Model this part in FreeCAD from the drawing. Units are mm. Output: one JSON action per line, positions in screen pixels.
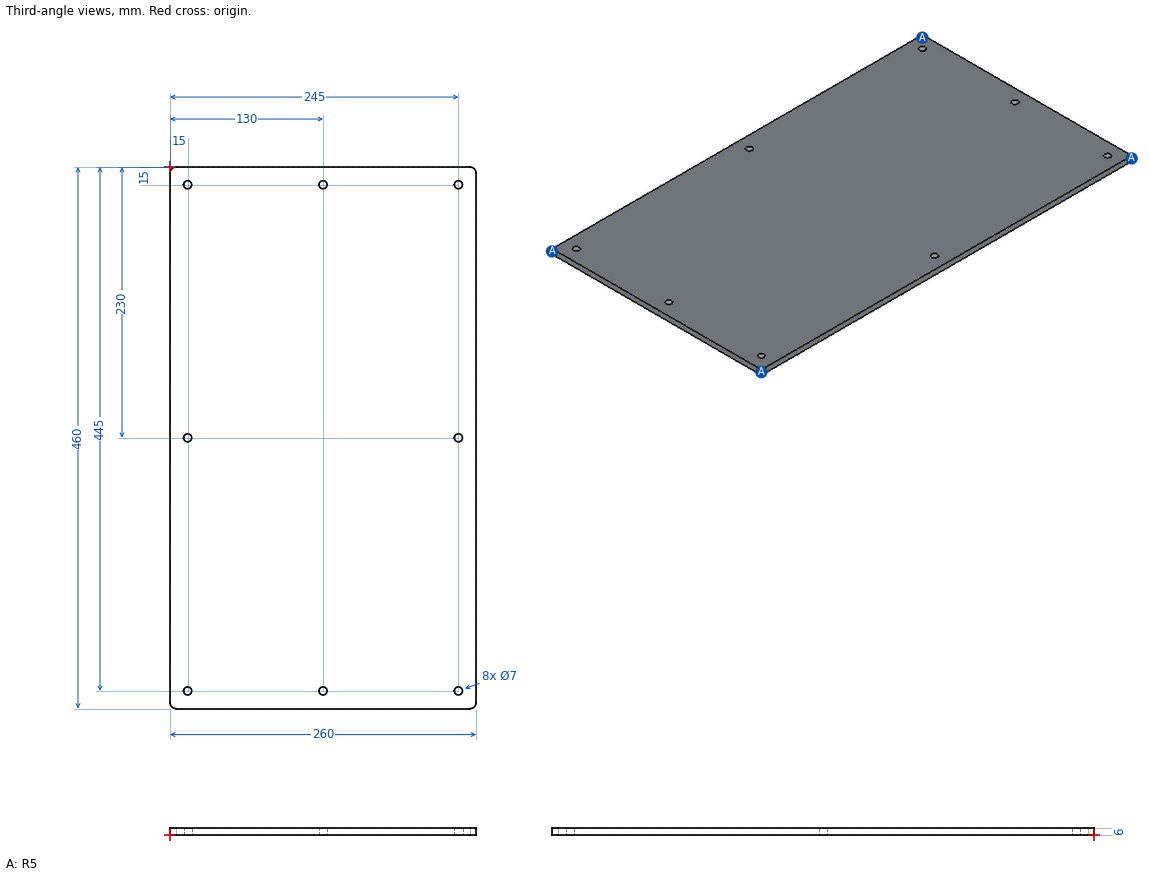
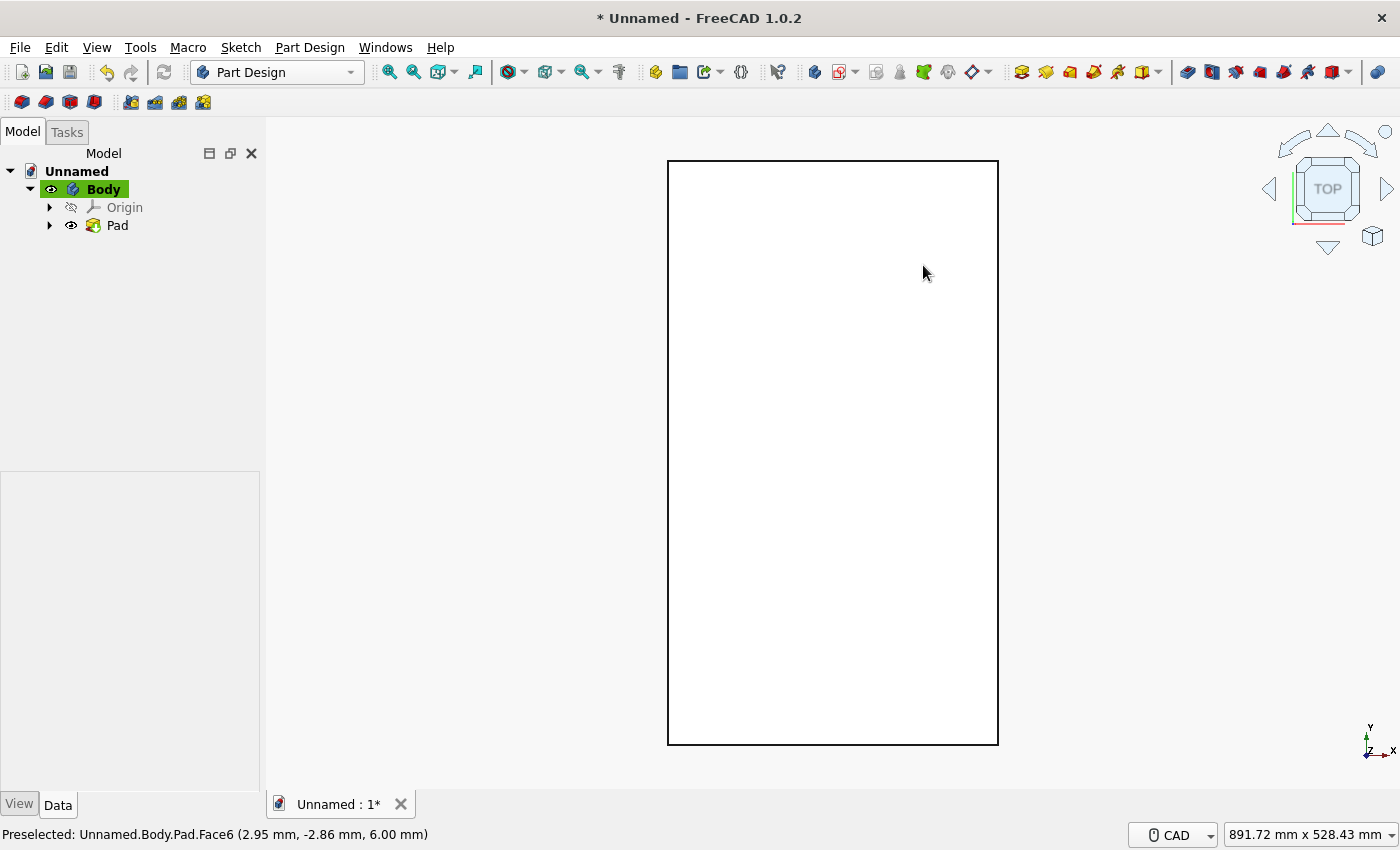
{"action": "scroll", "coordinate": [668, 160], "scroll_direction": "up", "scroll_amount": 9}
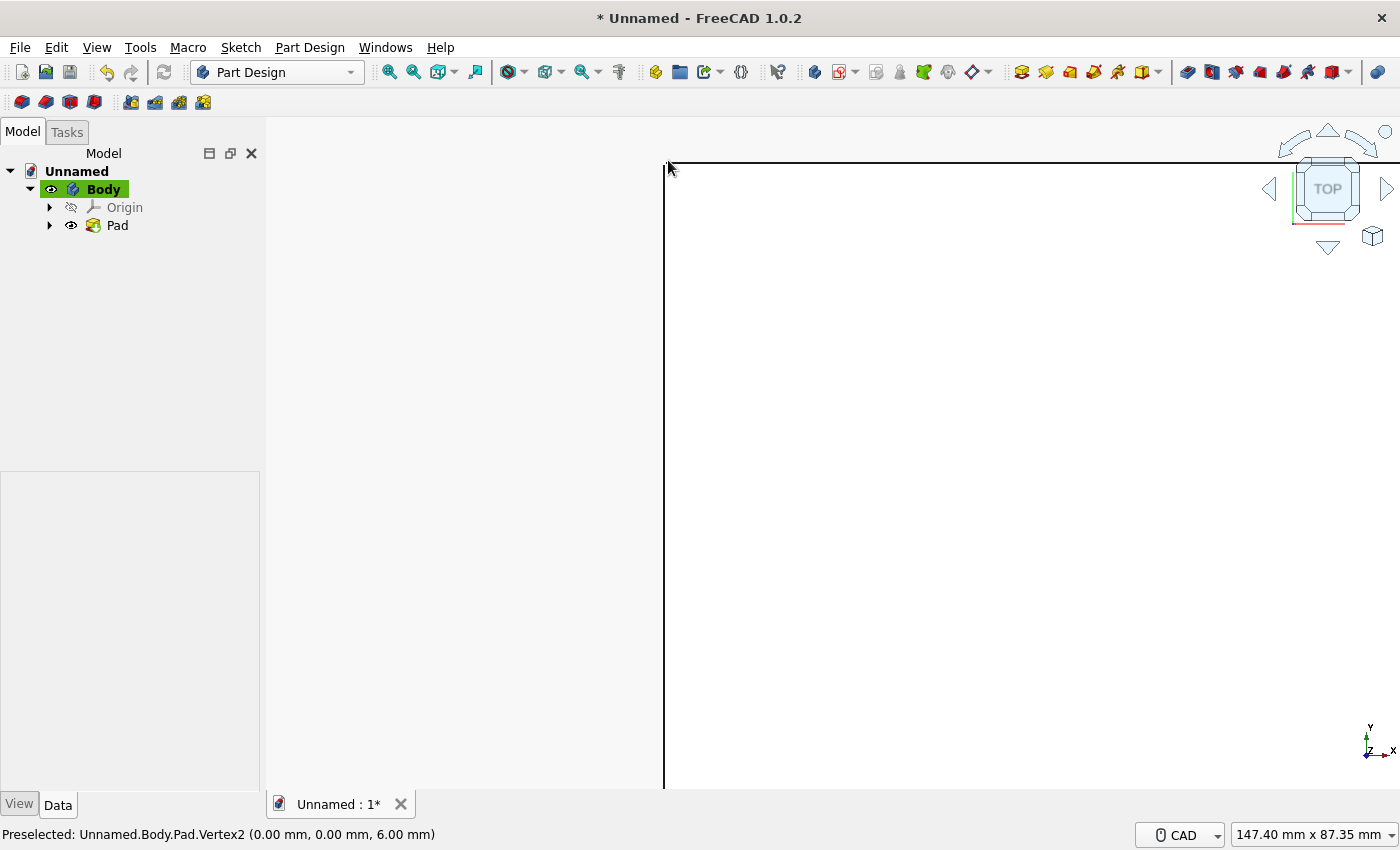
{"action": "key", "text": "v f"}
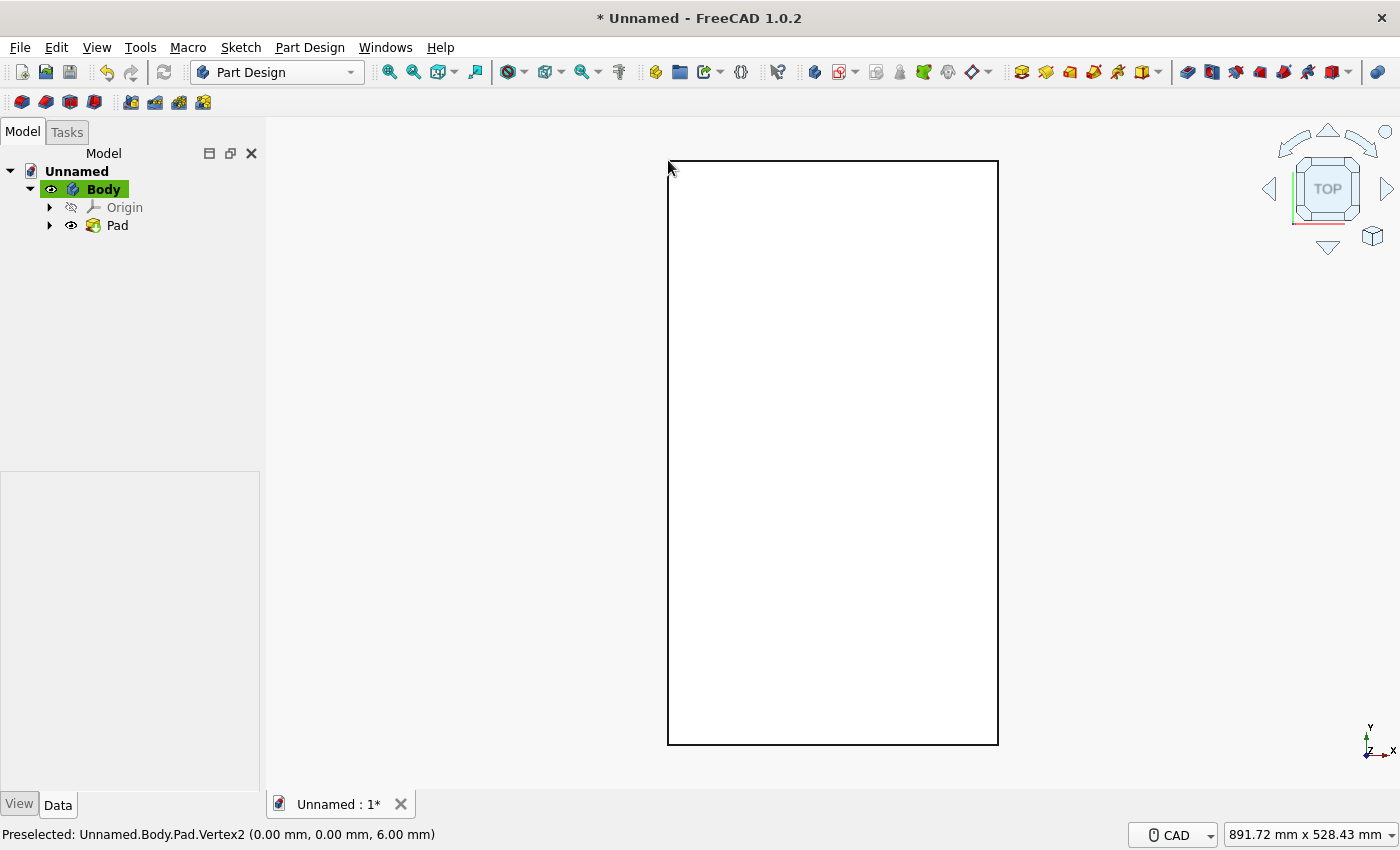
{"action": "key", "text": "1"}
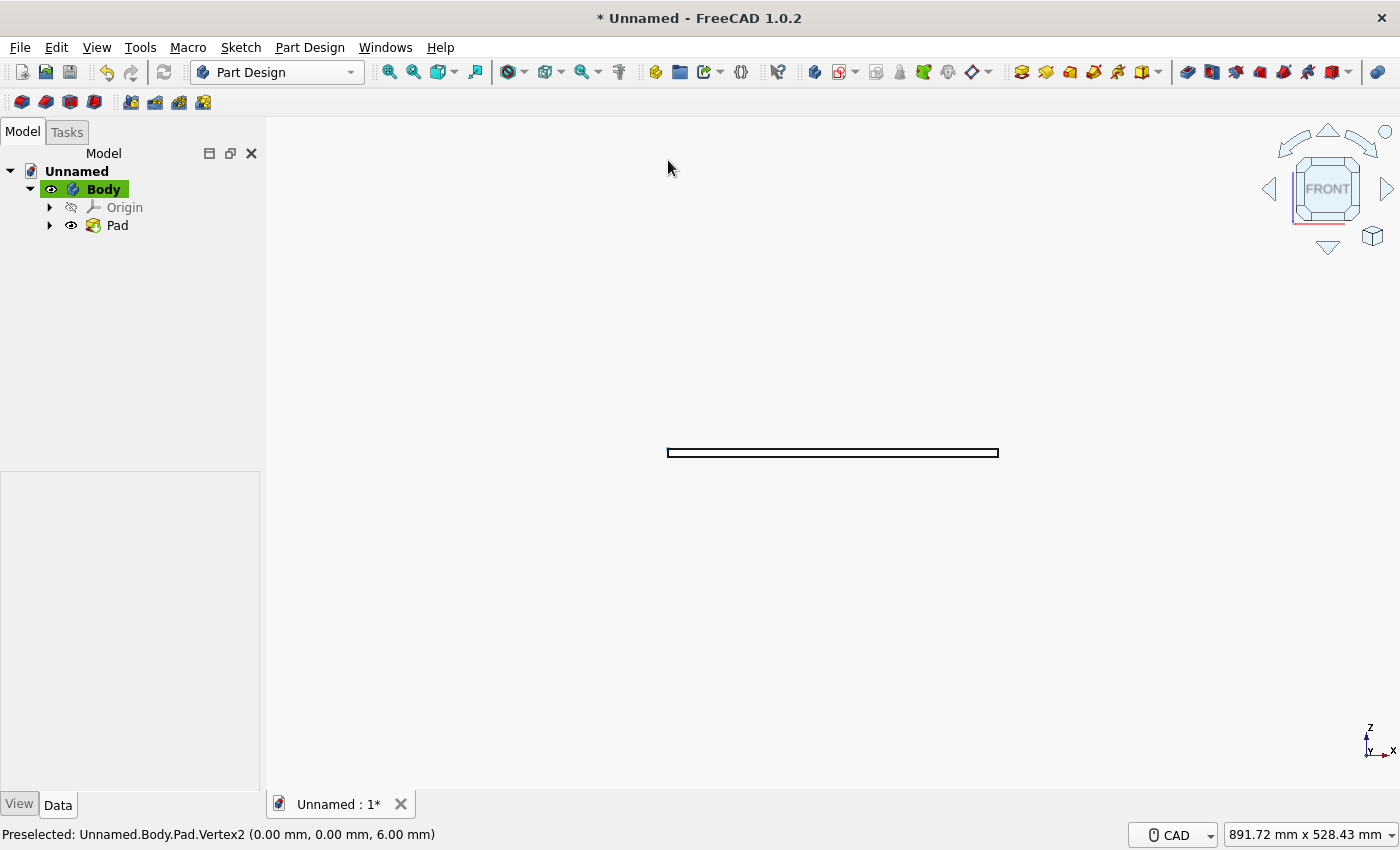
{"action": "key", "text": "v f"}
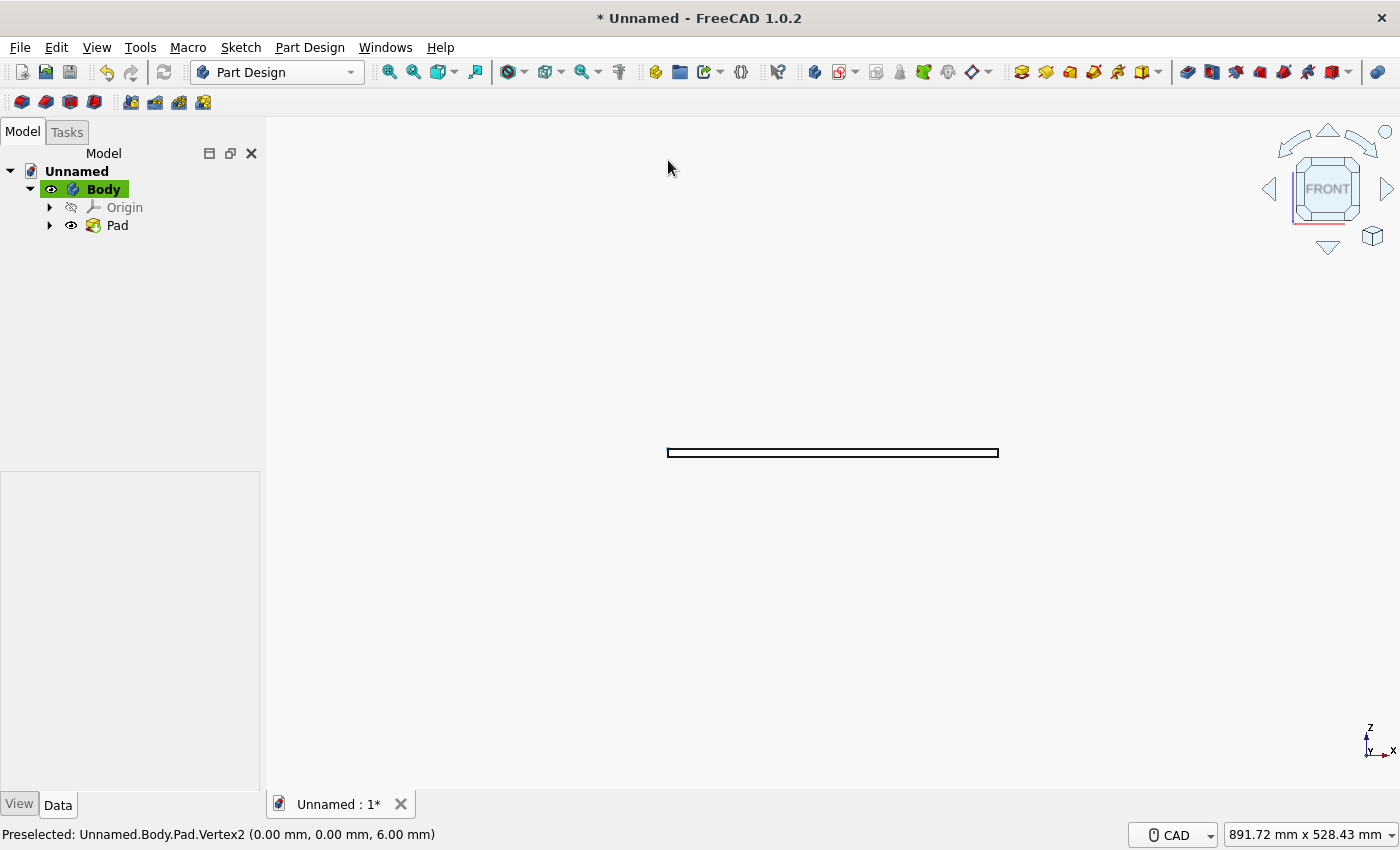
{"action": "scroll", "coordinate": [668, 452], "scroll_direction": "up", "scroll_amount": 9}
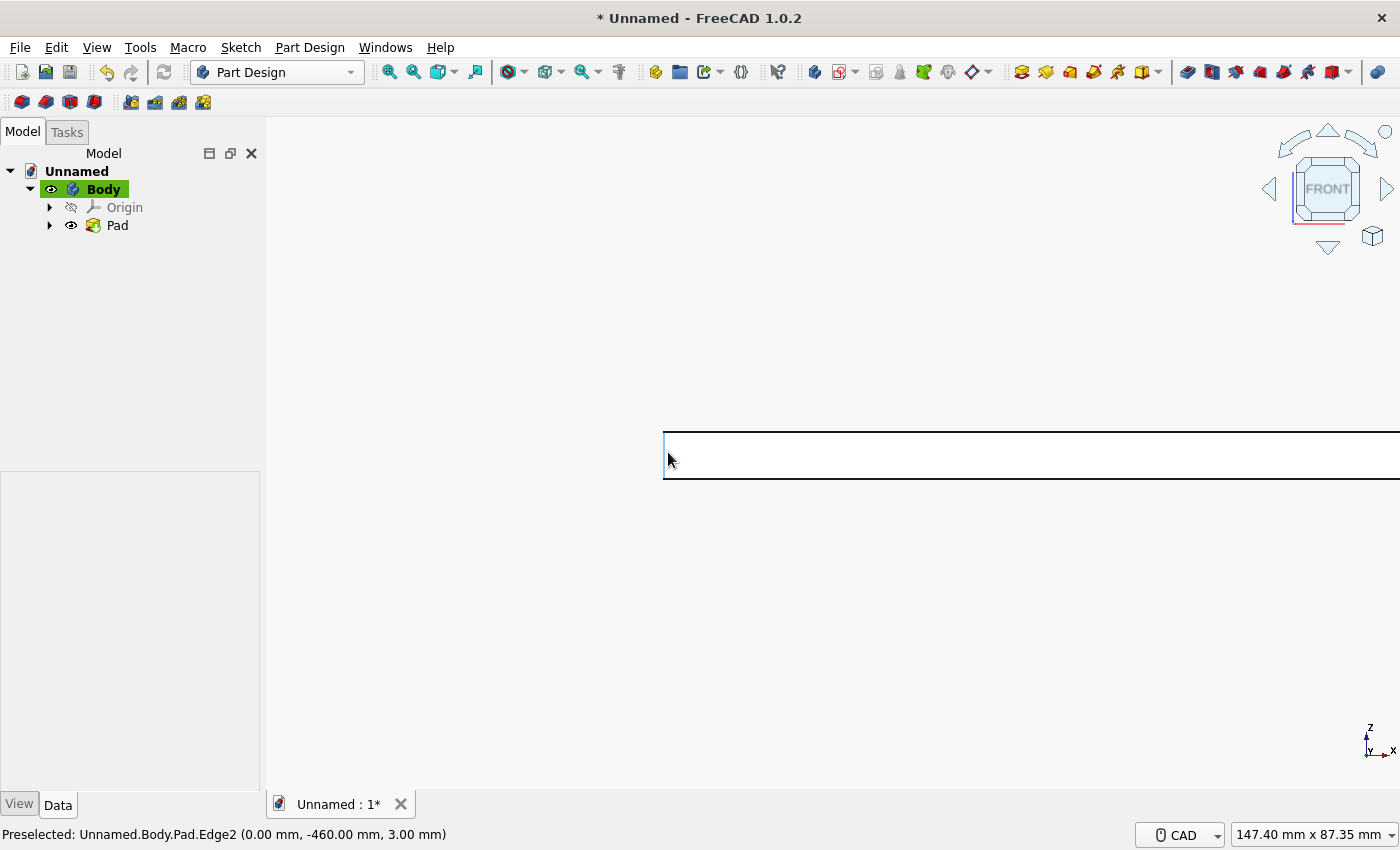
{"action": "left_click", "coordinate": [664, 455]}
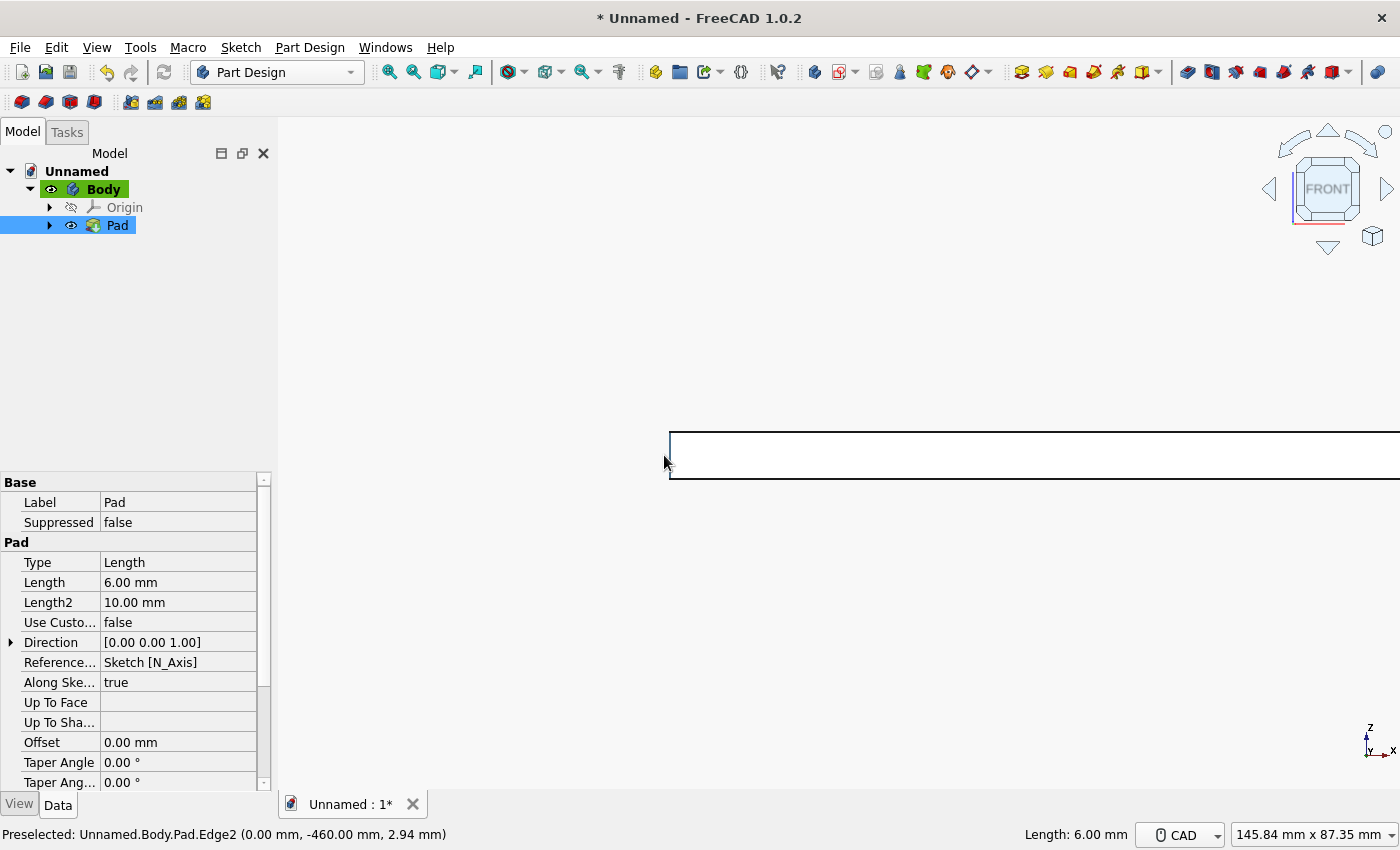
{"action": "key", "text": "v f"}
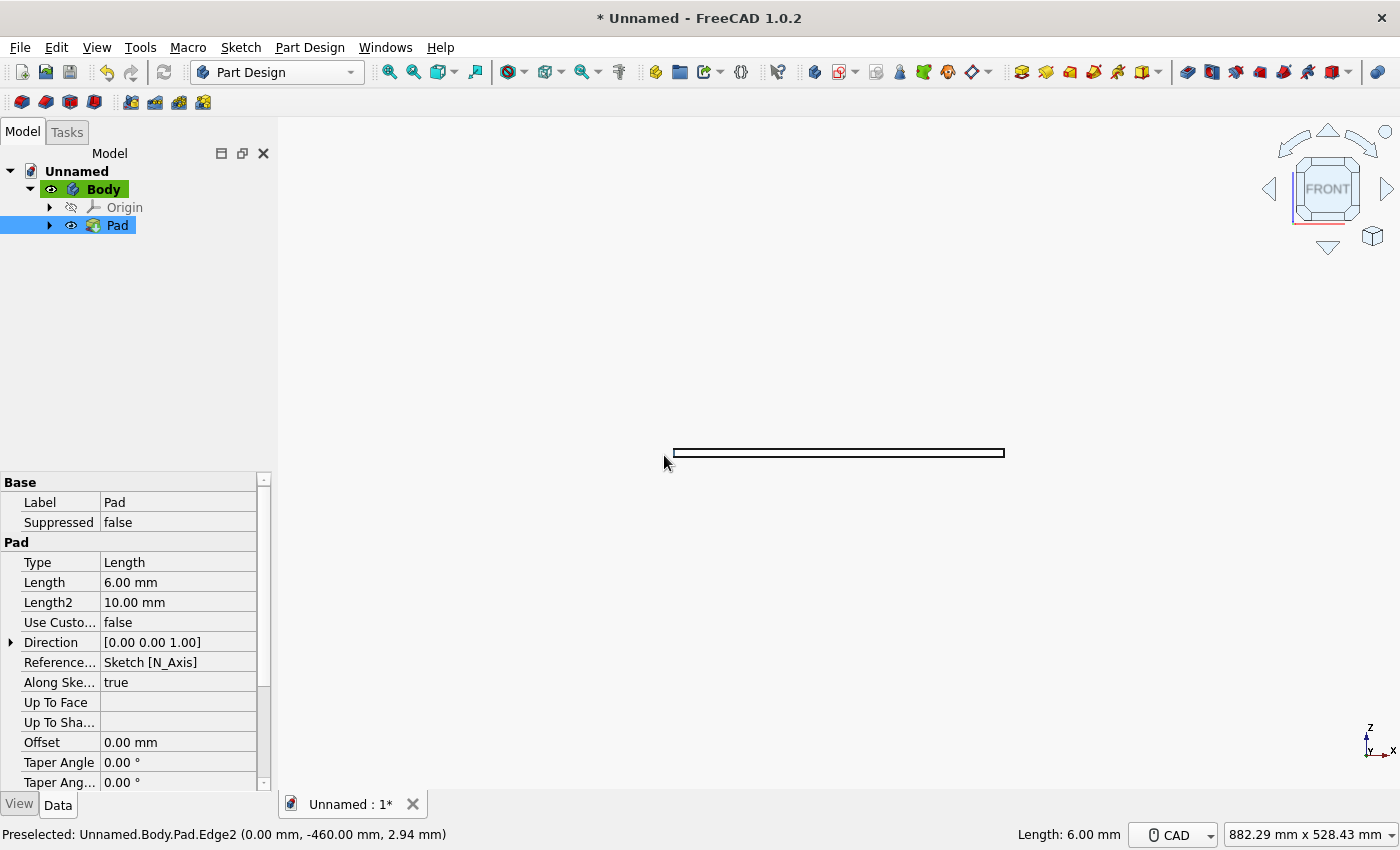
{"action": "key", "text": "3"}